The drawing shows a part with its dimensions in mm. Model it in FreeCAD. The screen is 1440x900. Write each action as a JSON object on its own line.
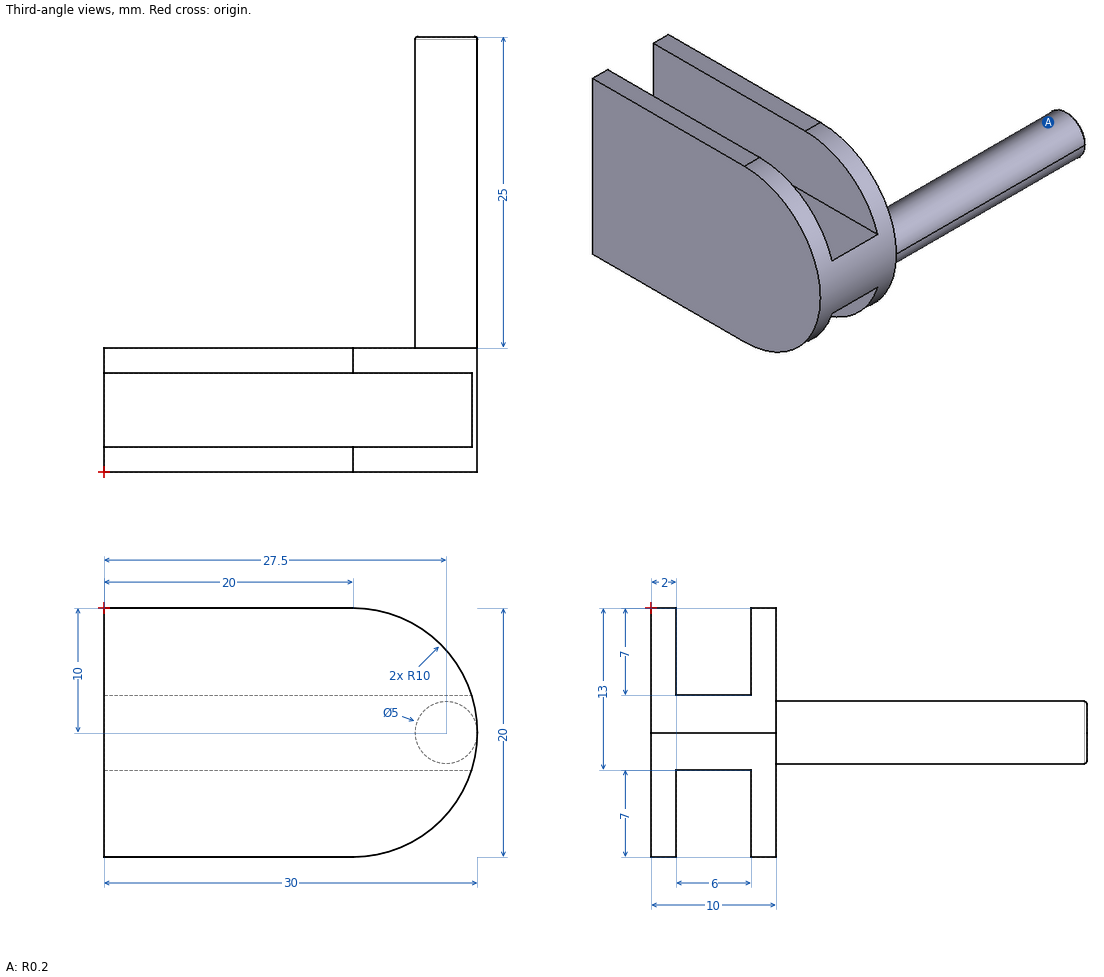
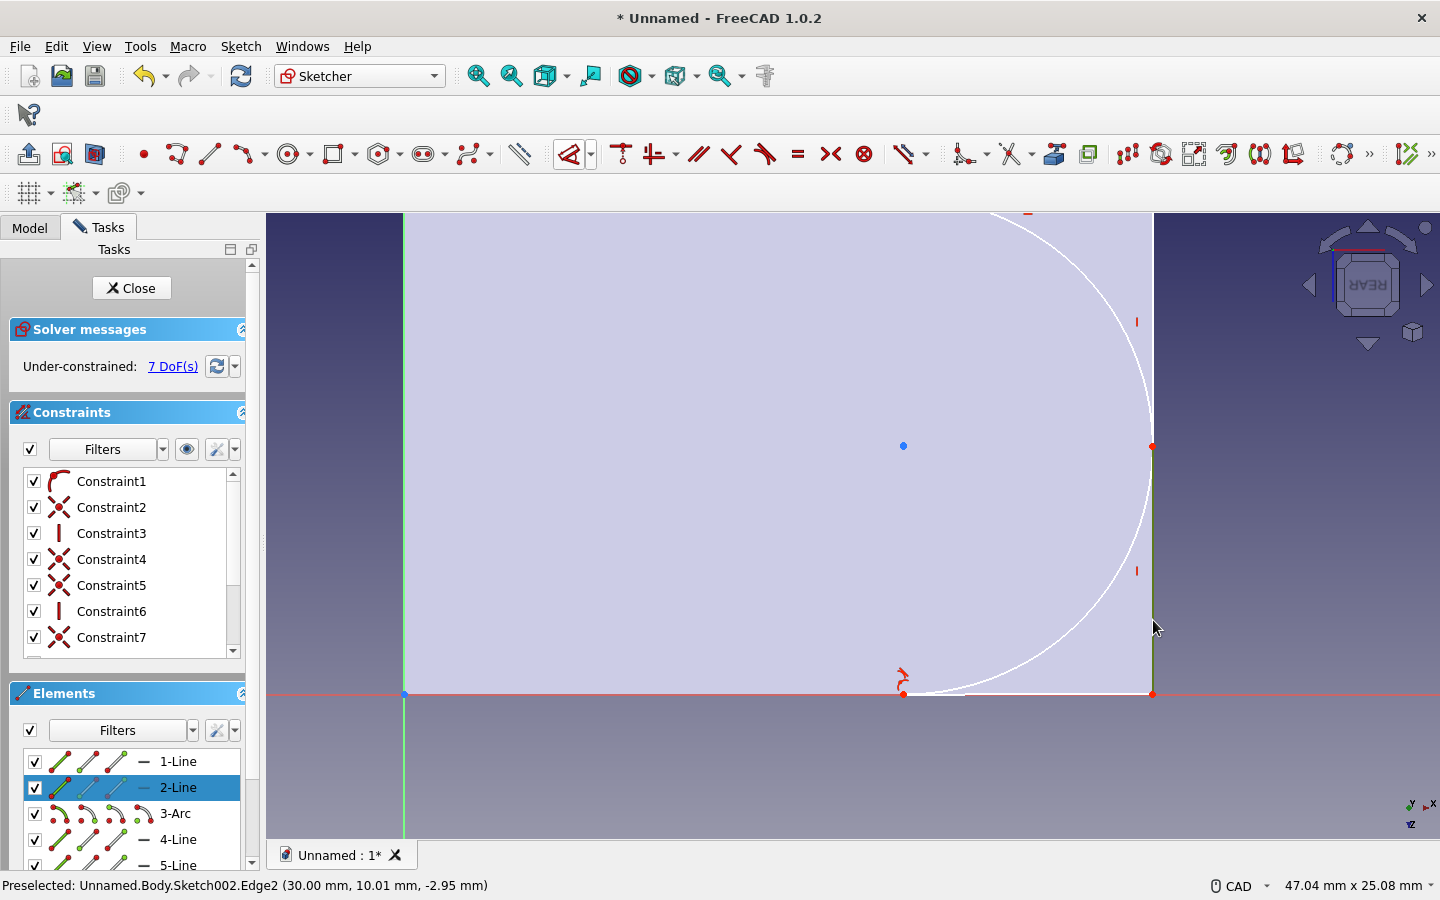
{"action": "left_click", "coordinate": [1017, 667]}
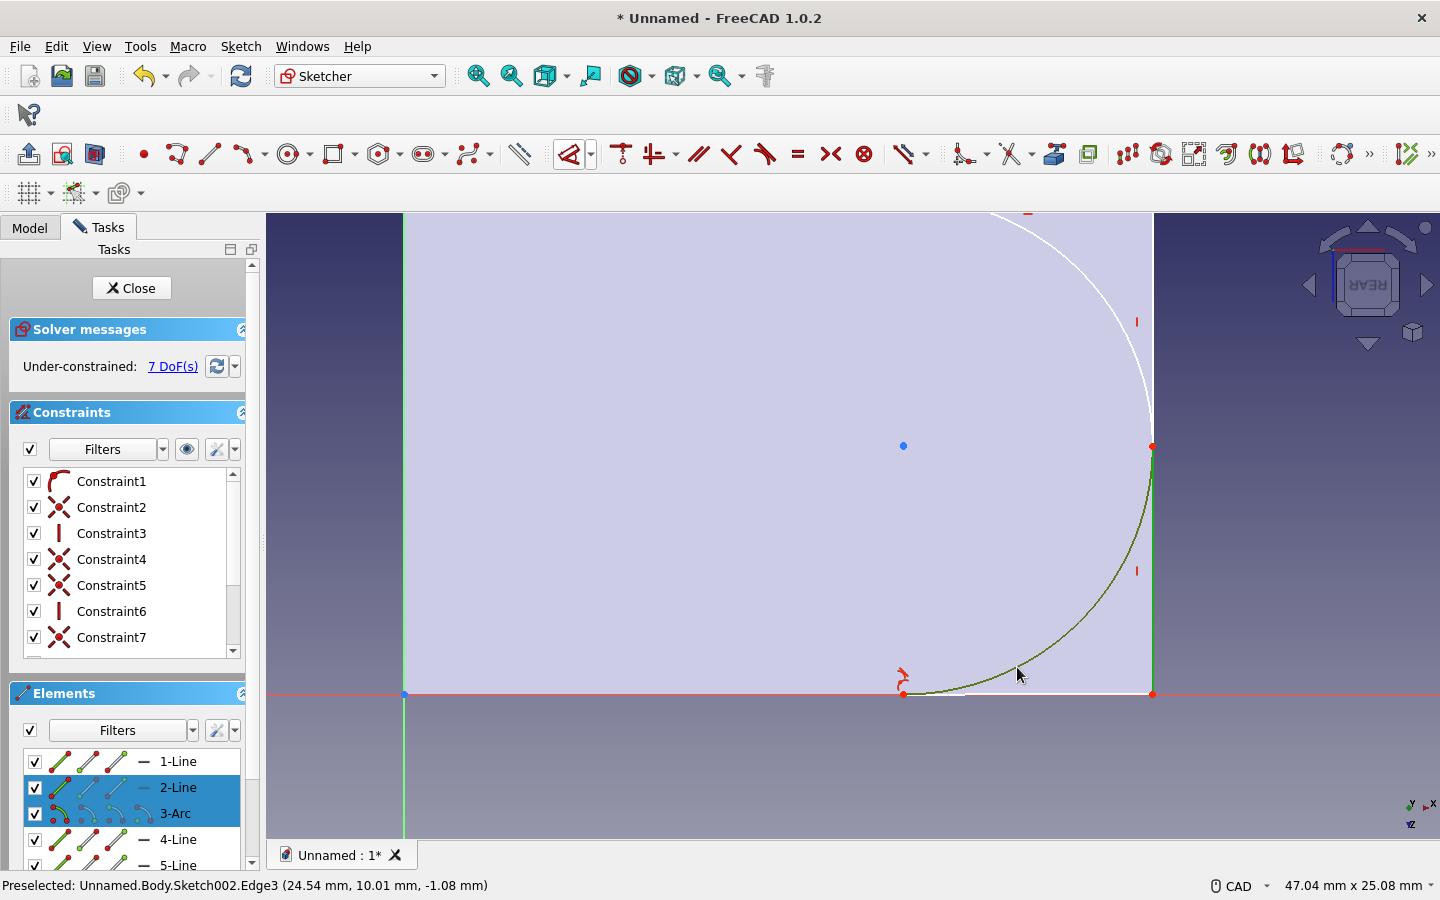
{"action": "left_click", "coordinate": [765, 154]}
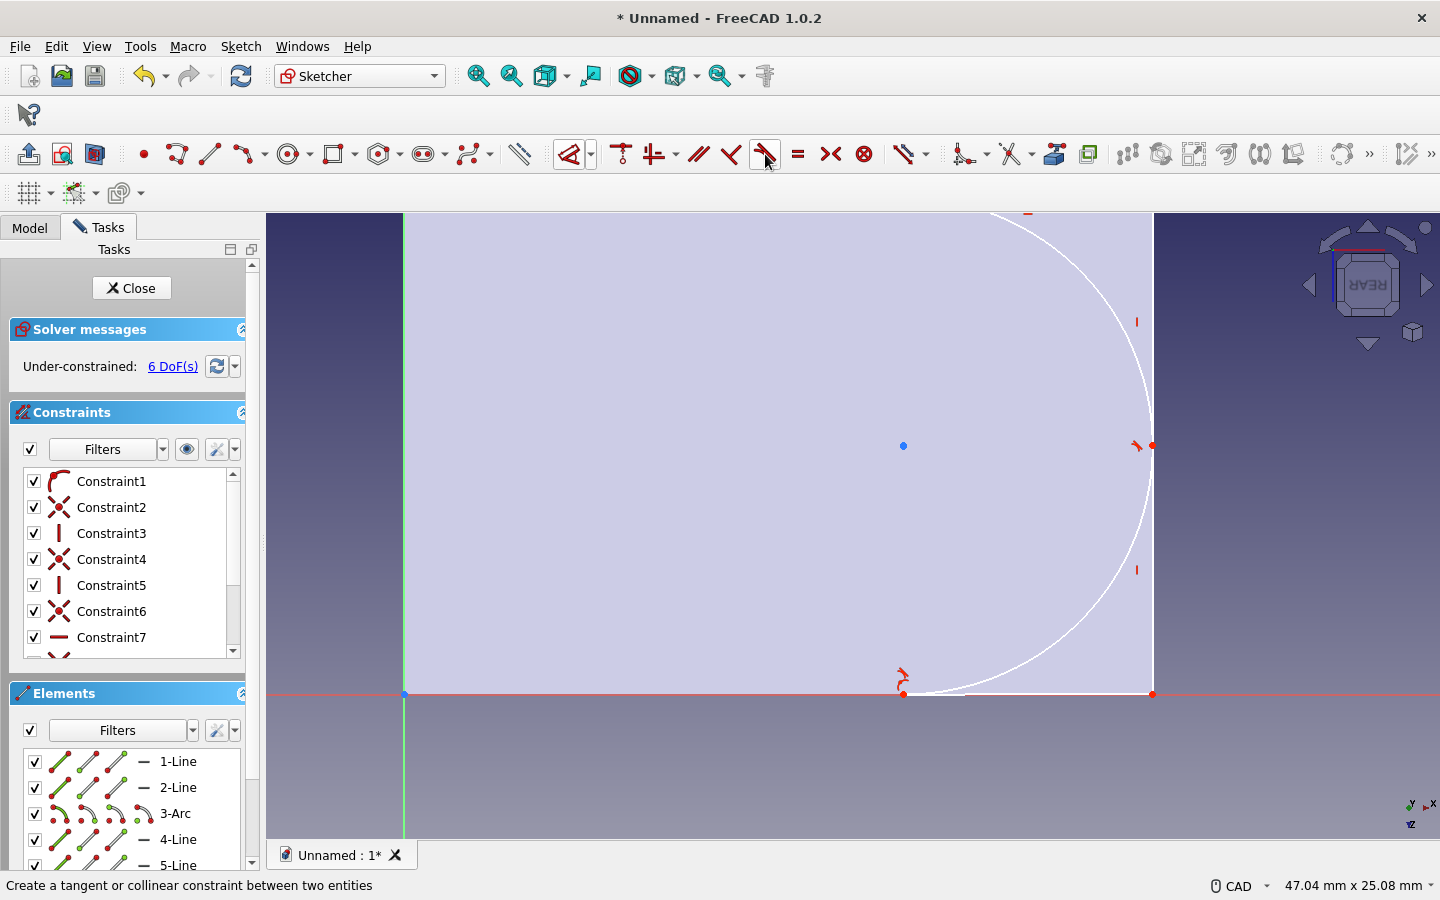
{"action": "left_click", "coordinate": [1153, 620]}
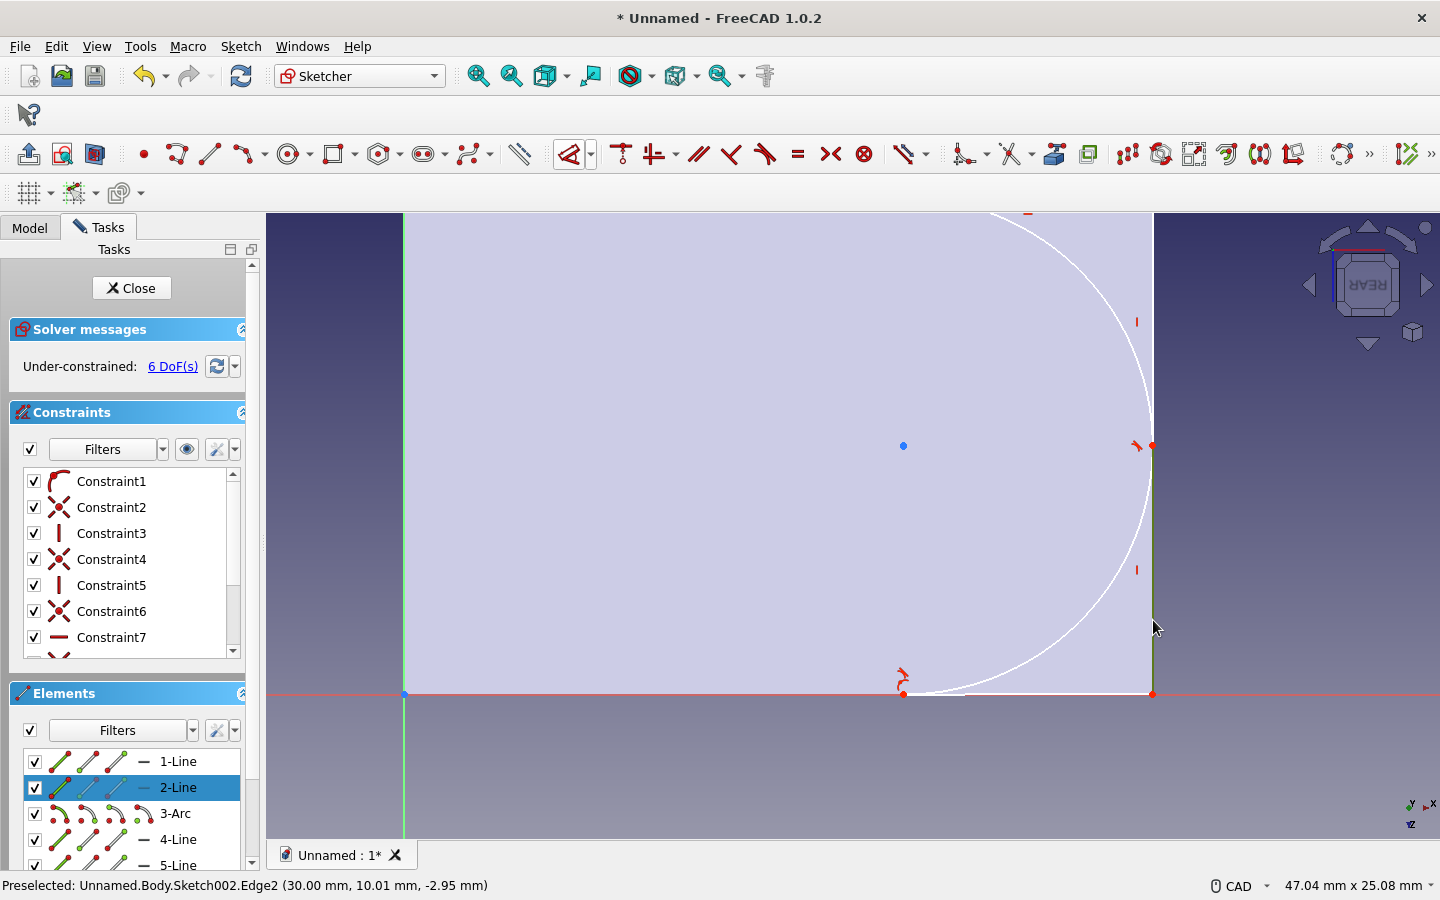
{"action": "left_click", "coordinate": [1125, 333]}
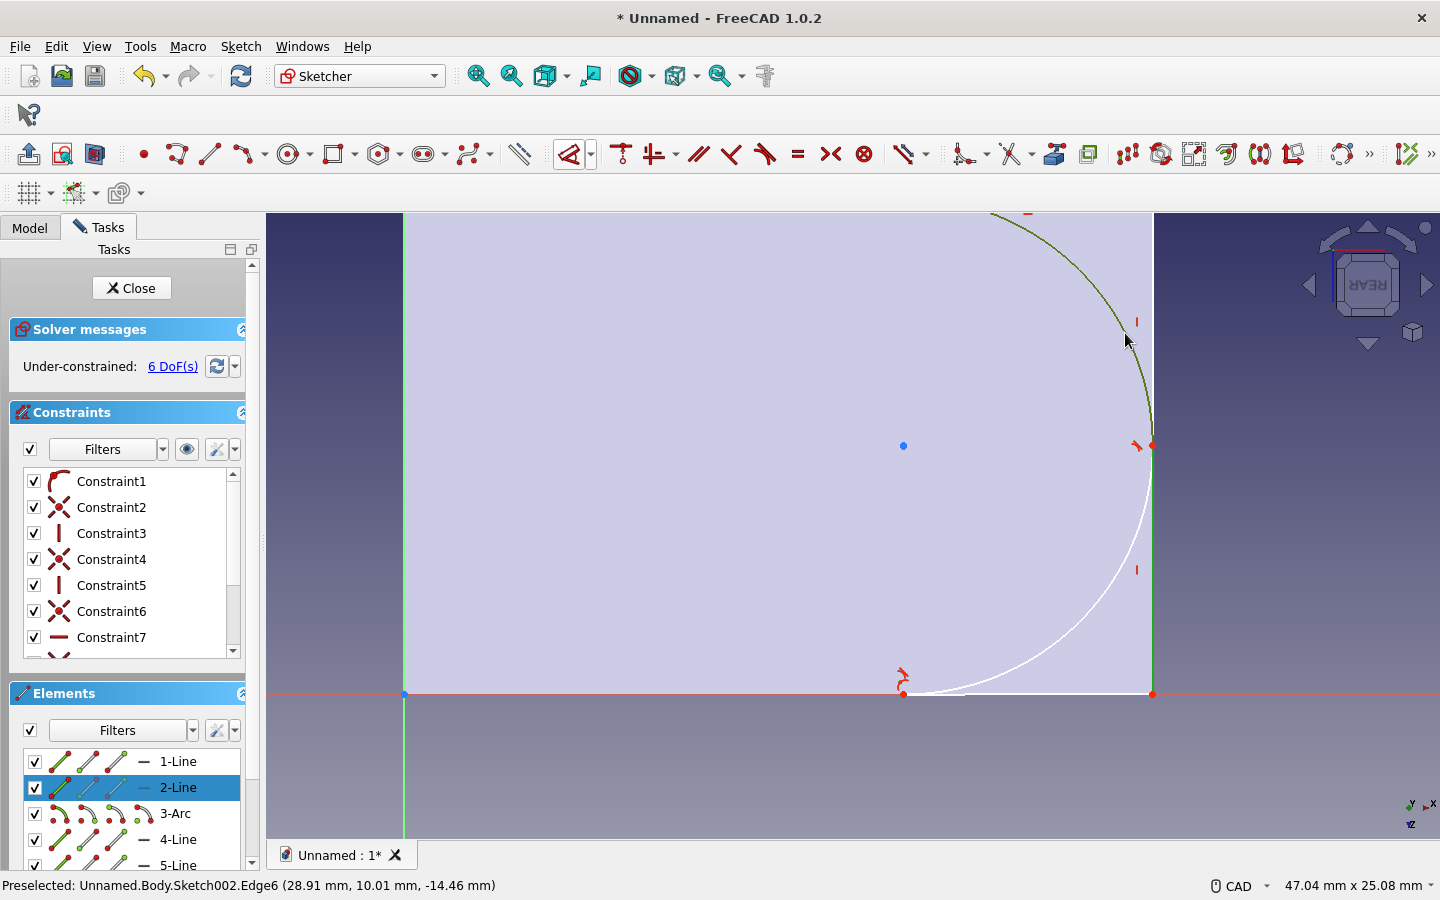
{"action": "left_click", "coordinate": [765, 154]}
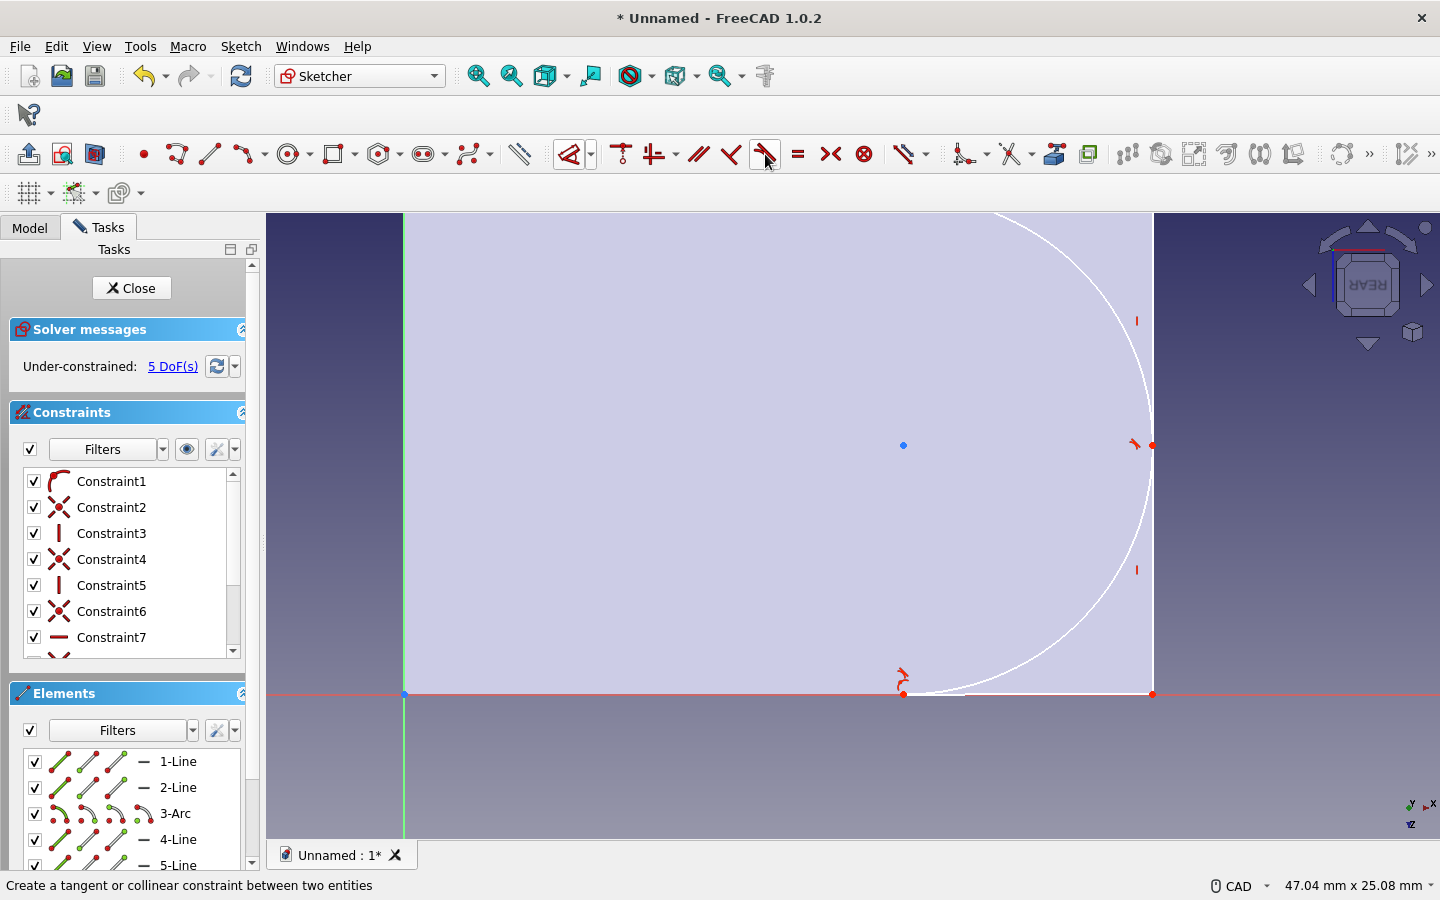
{"action": "scroll", "coordinate": [812, 811], "scroll_direction": "down", "scroll_amount": 1}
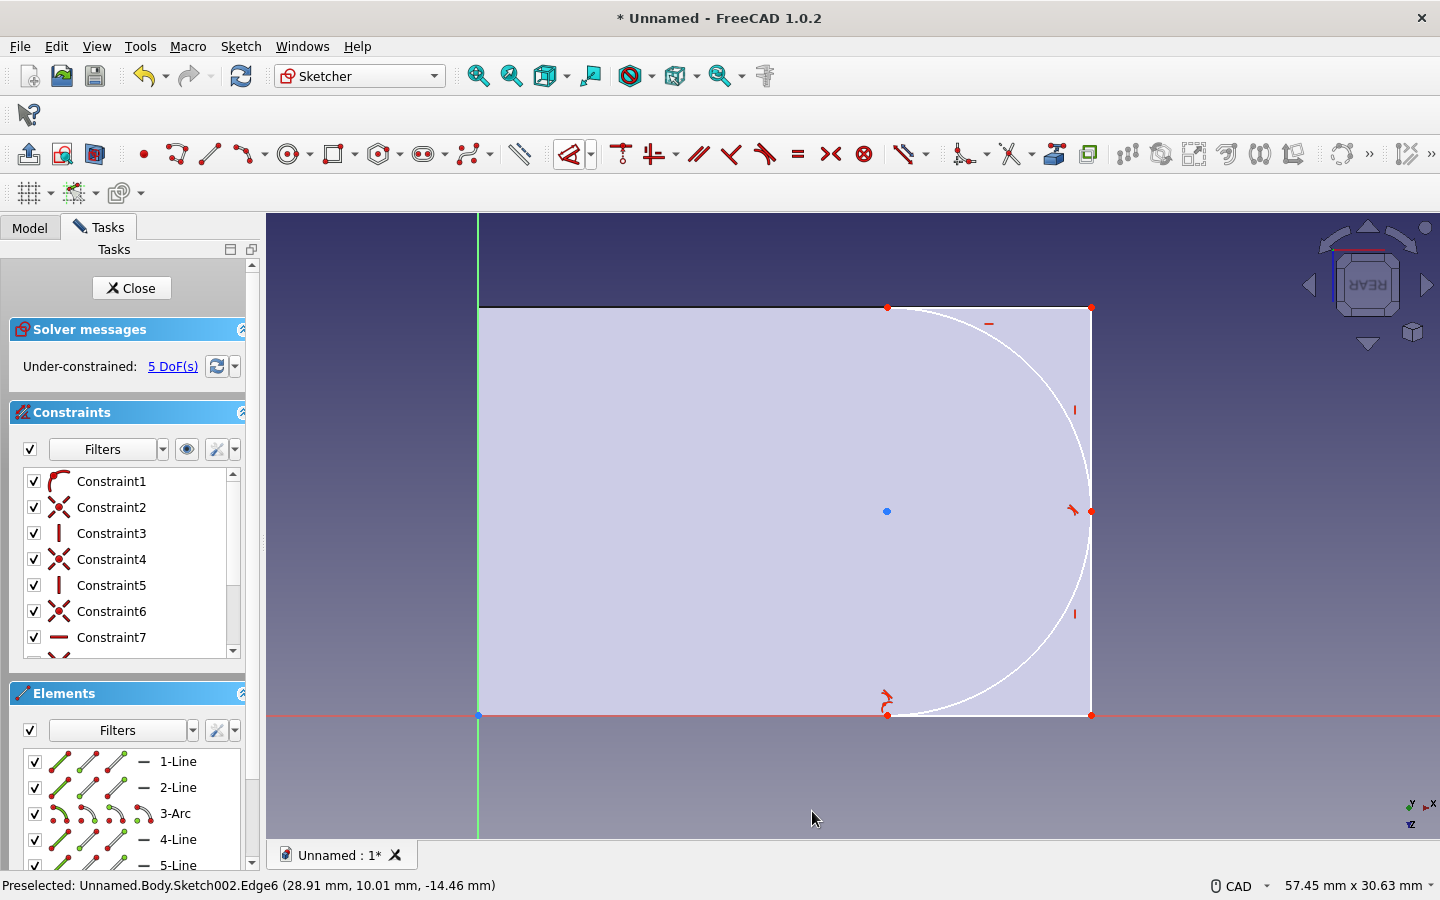
{"action": "left_click", "coordinate": [1030, 308]}